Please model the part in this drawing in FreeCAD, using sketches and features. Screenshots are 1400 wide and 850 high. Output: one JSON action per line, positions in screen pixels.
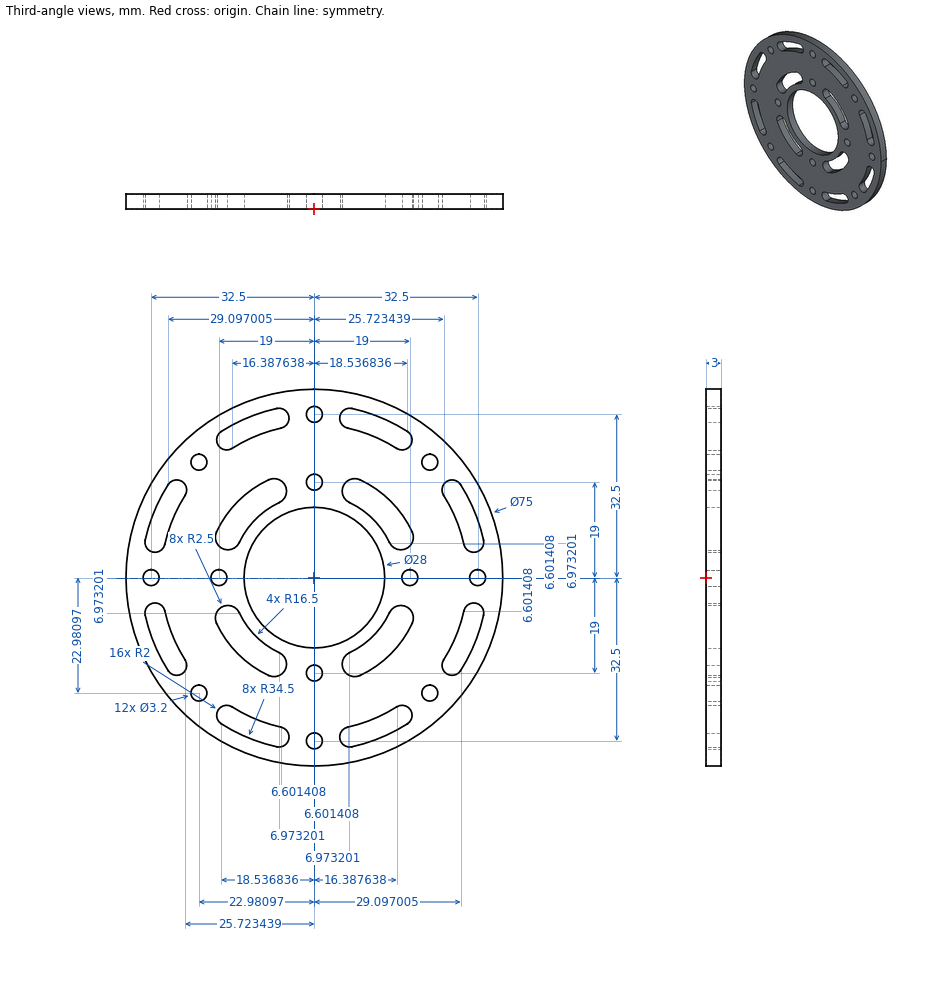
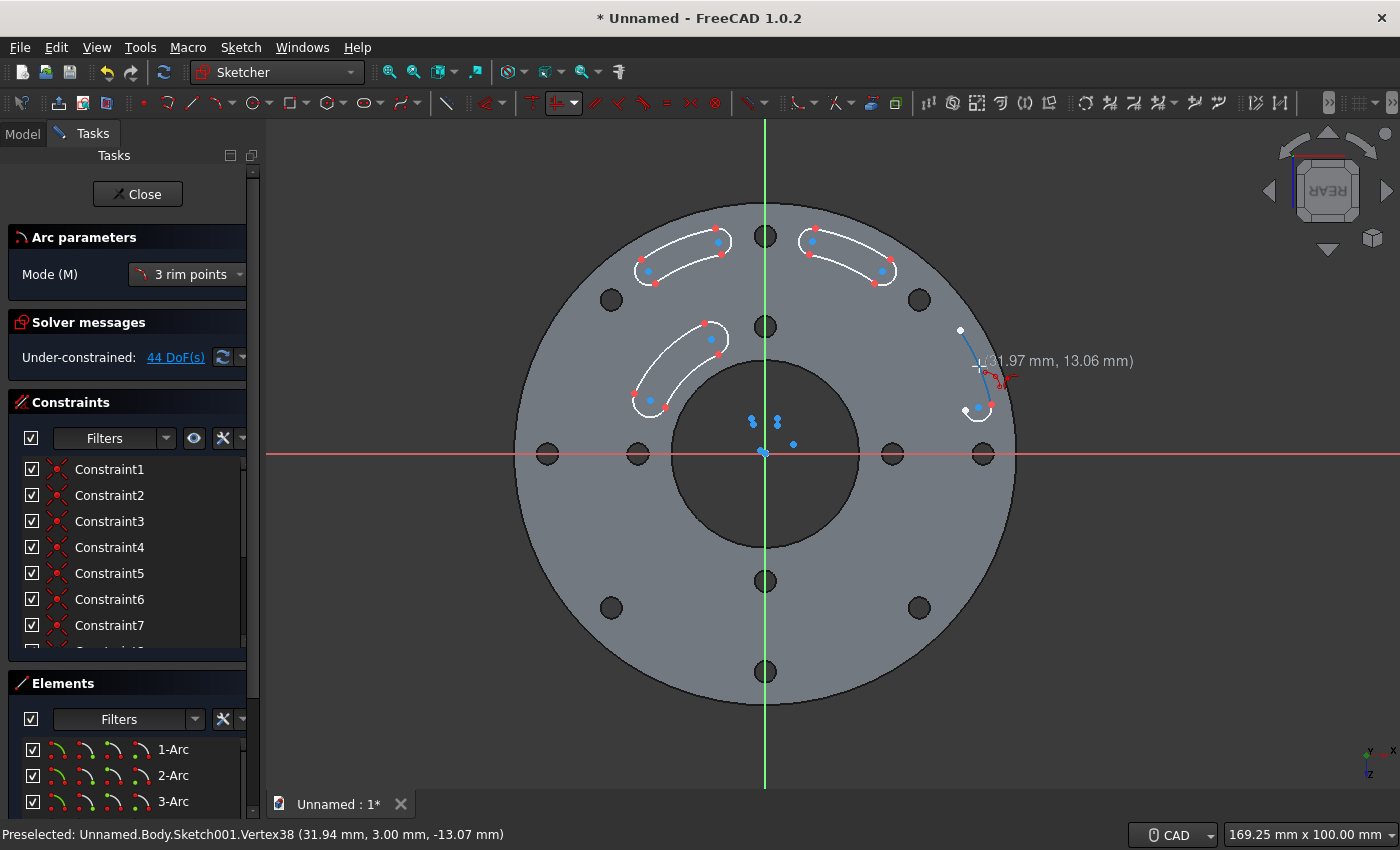
{"action": "left_click", "coordinate": [960, 331]}
{"action": "left_click", "coordinate": [938, 344]}
{"action": "left_click", "coordinate": [942, 326]}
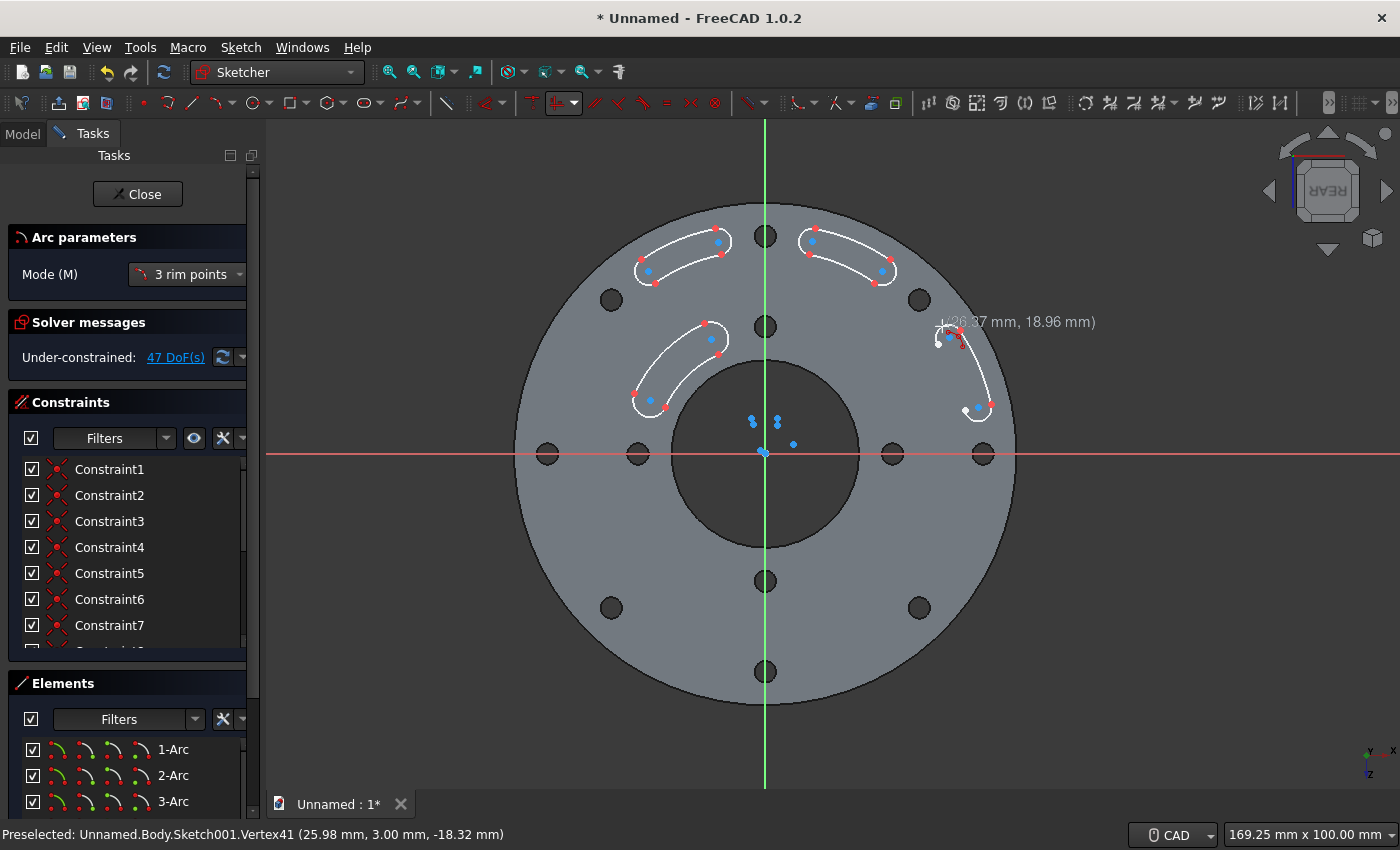
{"action": "left_click", "coordinate": [938, 345]}
{"action": "left_click", "coordinate": [965, 411]}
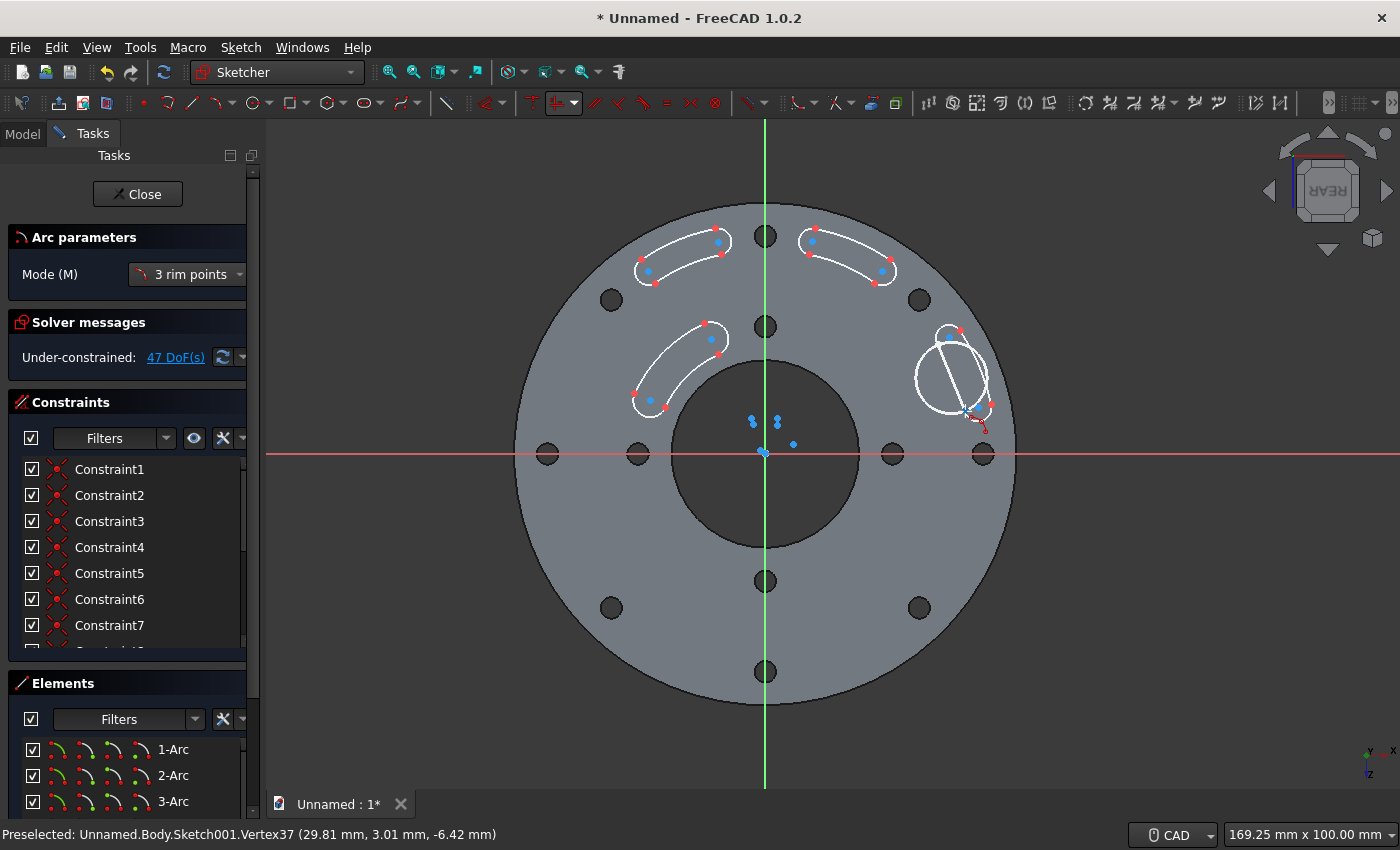
{"action": "scroll", "coordinate": [954, 376], "scroll_direction": "up", "scroll_amount": 9}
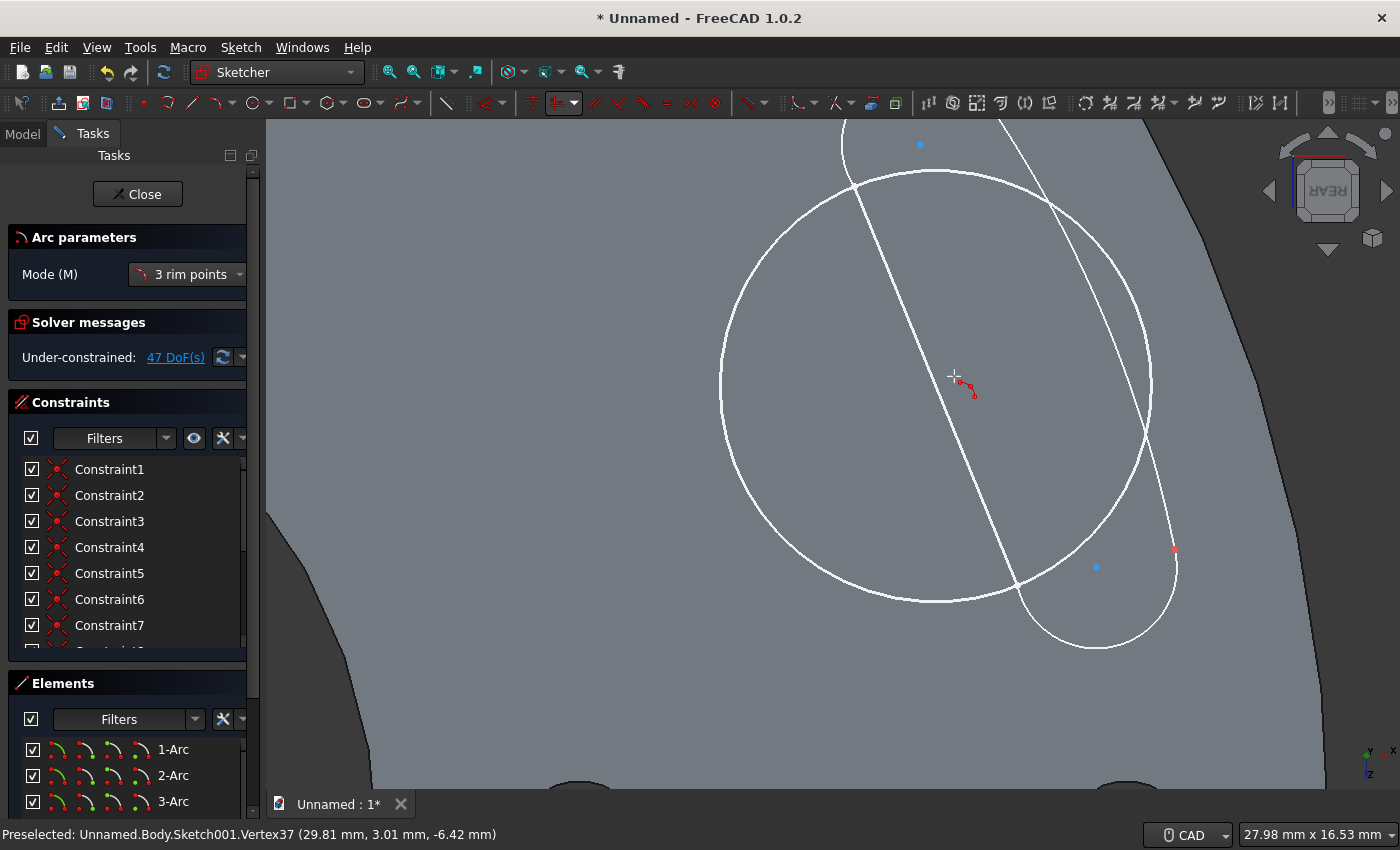
{"action": "left_click", "coordinate": [952, 373]}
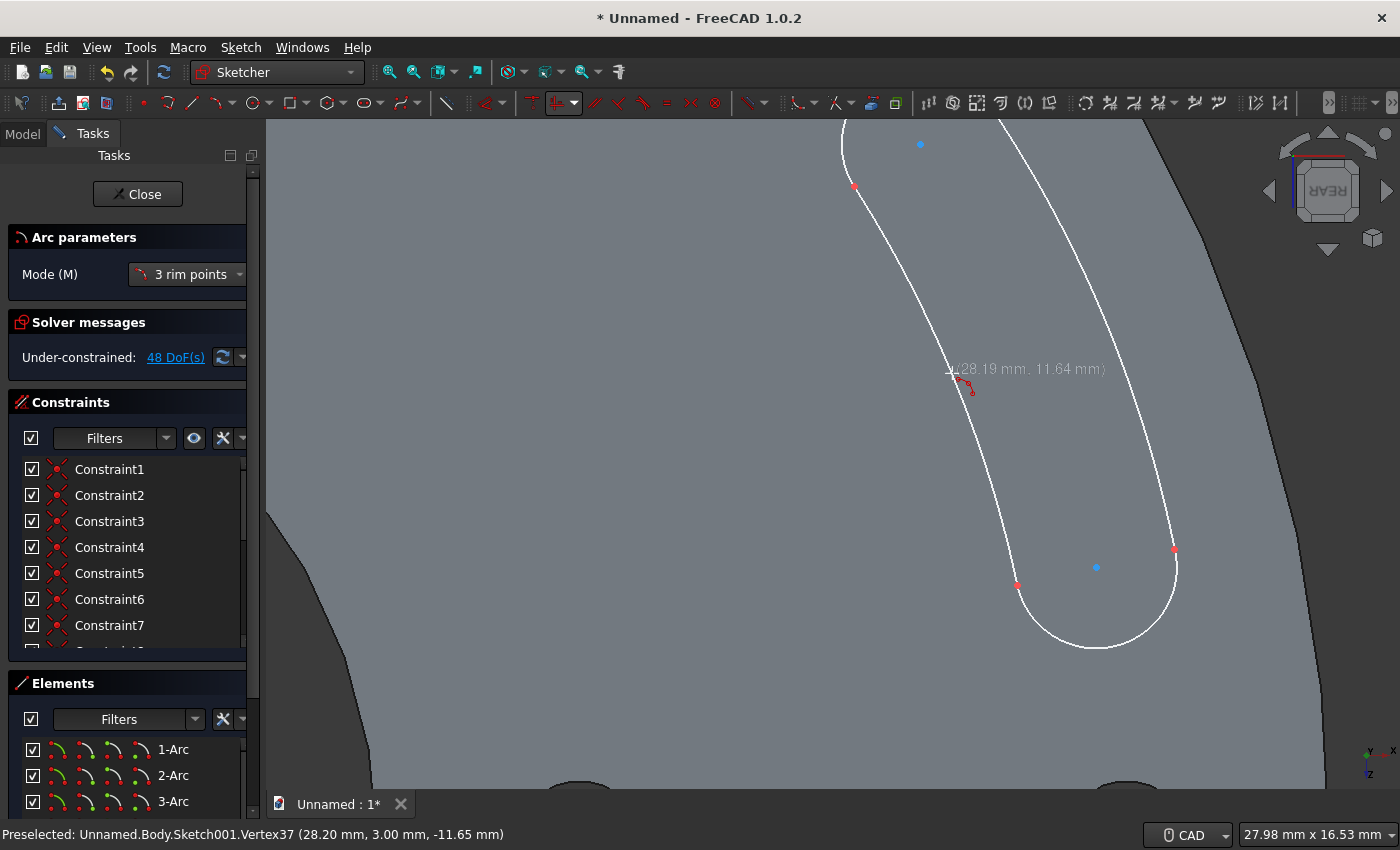
{"action": "scroll", "coordinate": [954, 376], "scroll_direction": "down", "scroll_amount": 9}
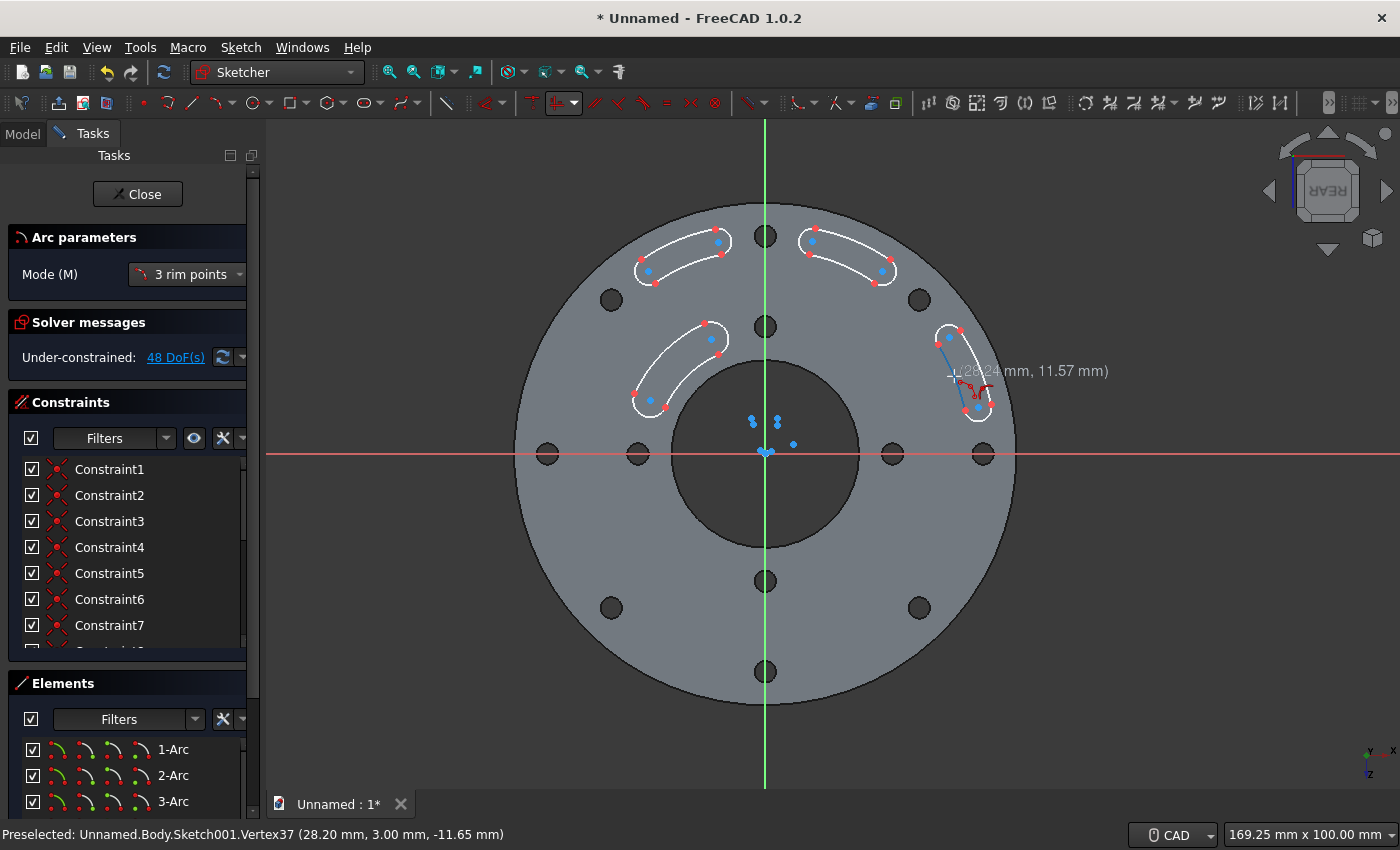
{"action": "left_click", "coordinate": [965, 498]}
{"action": "left_click", "coordinate": [938, 564]}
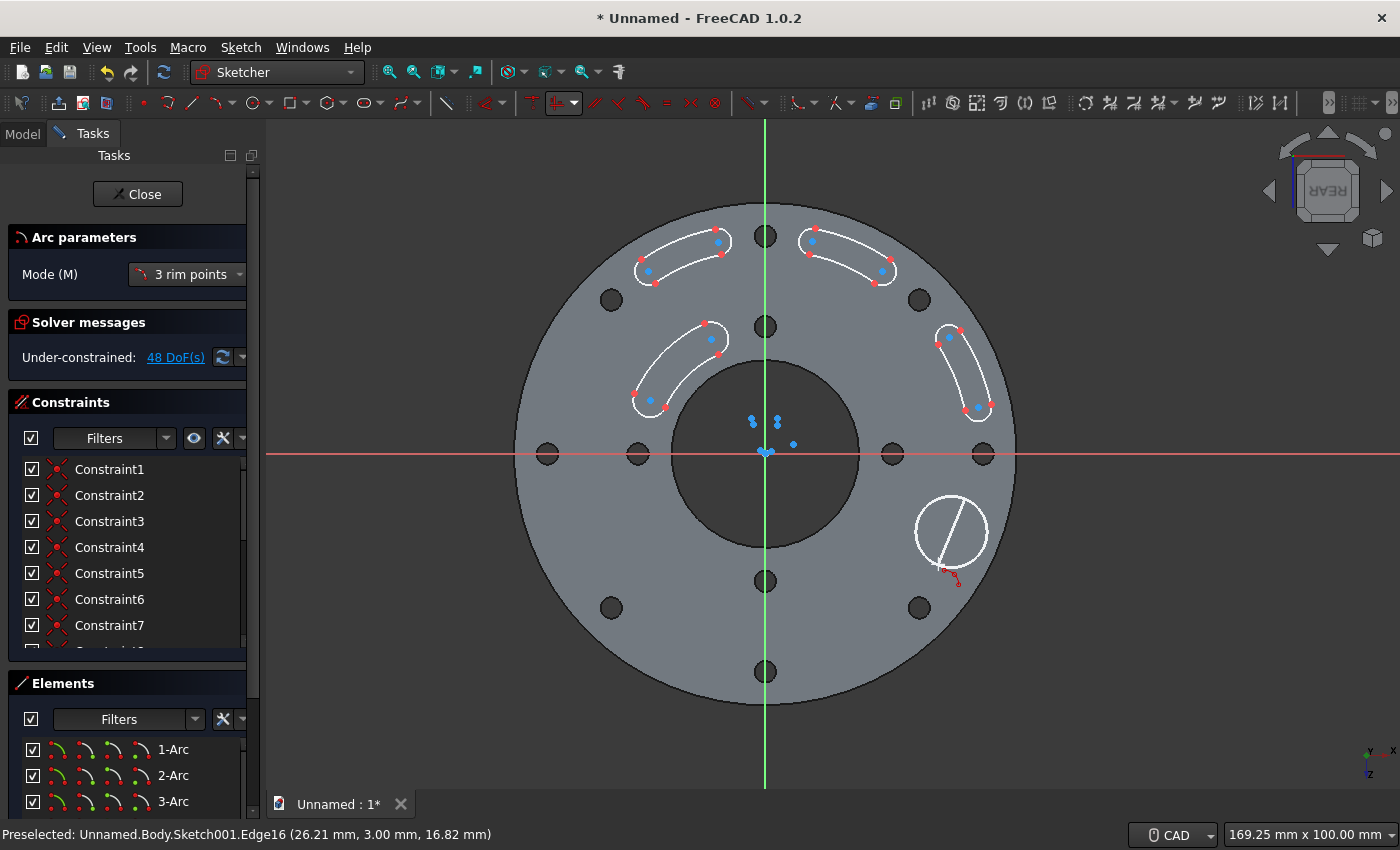
{"action": "scroll", "coordinate": [954, 532], "scroll_direction": "up", "scroll_amount": 9}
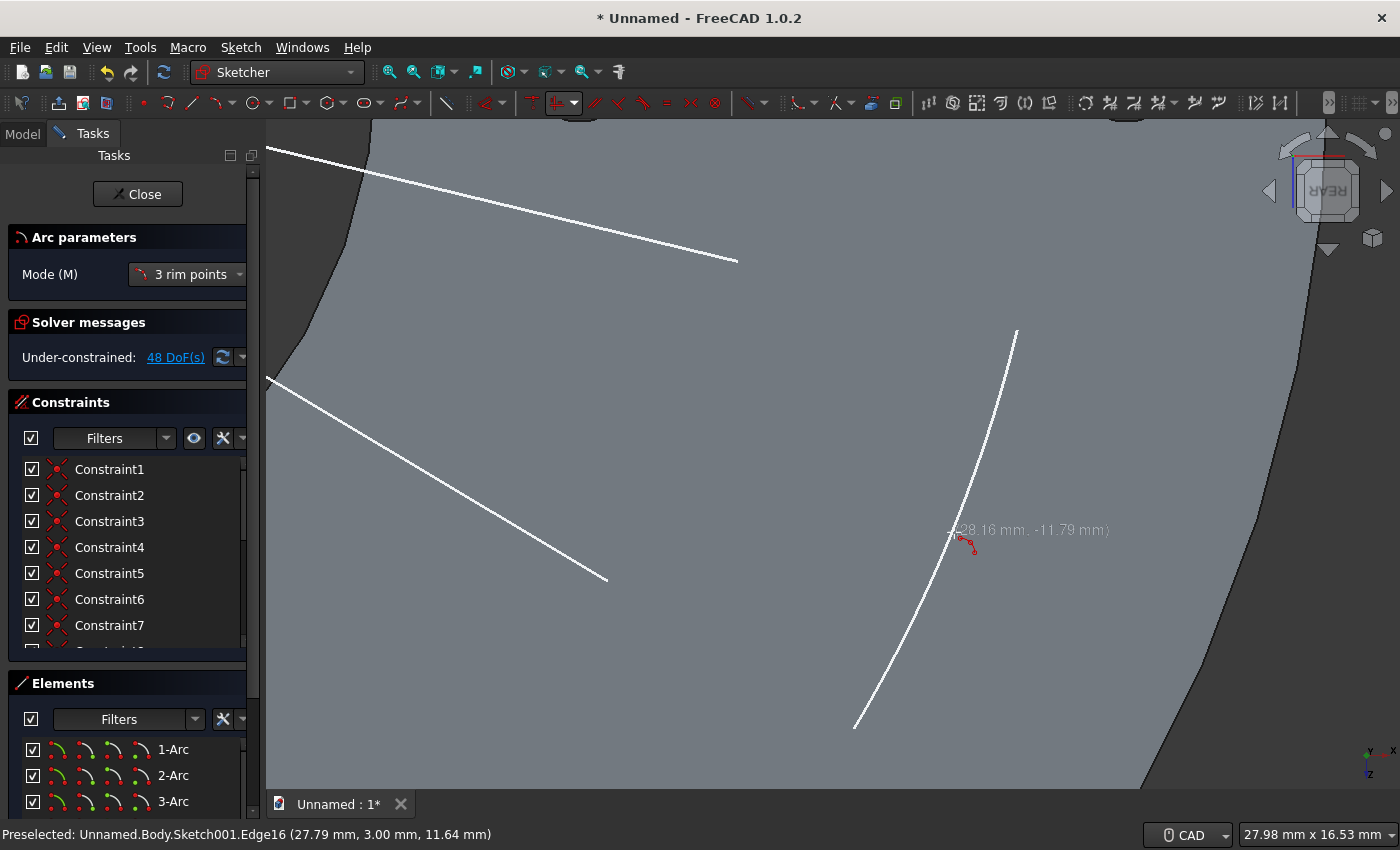
{"action": "left_click", "coordinate": [952, 530]}